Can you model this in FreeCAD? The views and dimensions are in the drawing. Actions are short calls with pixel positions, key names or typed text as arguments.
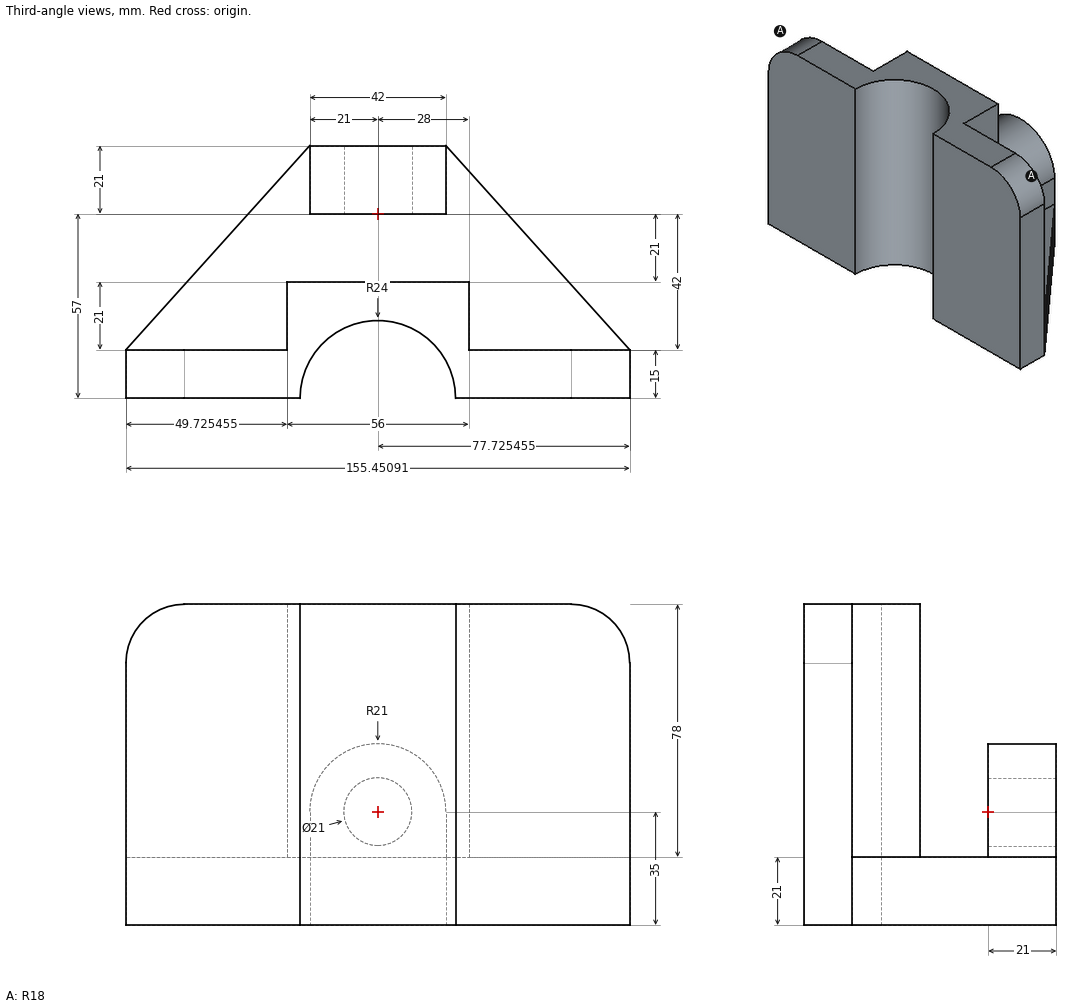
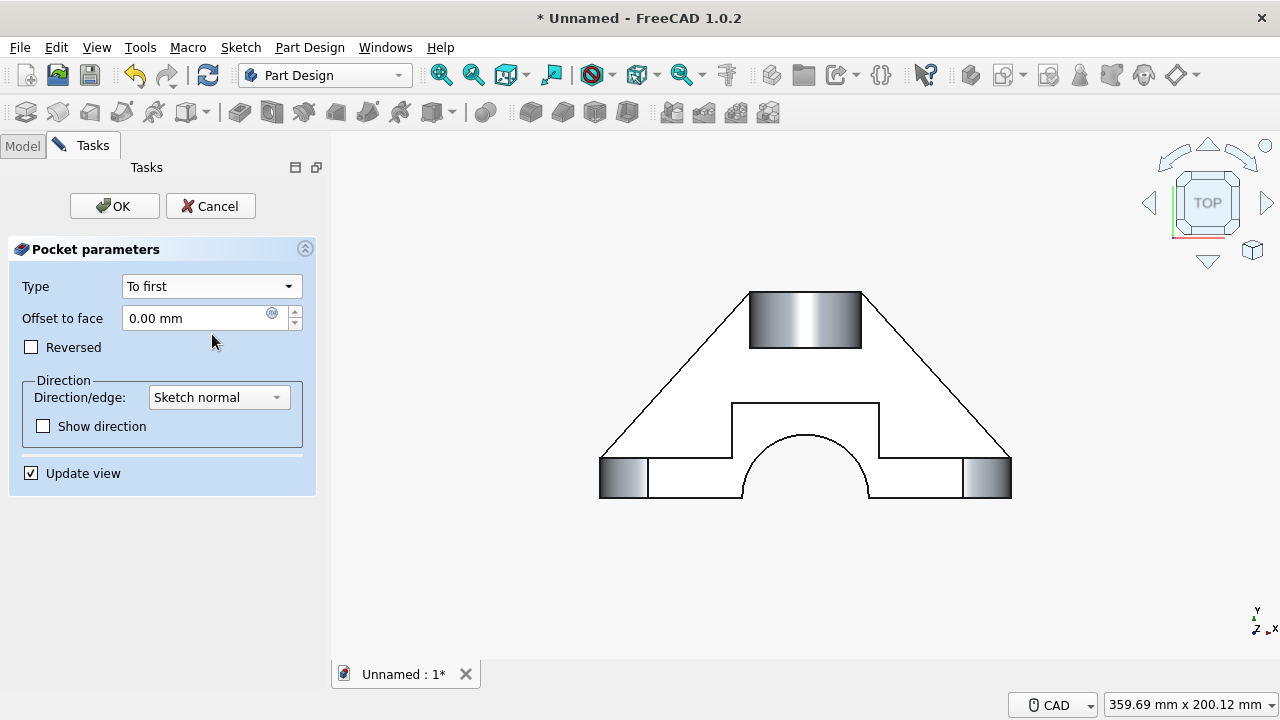
click(115, 206)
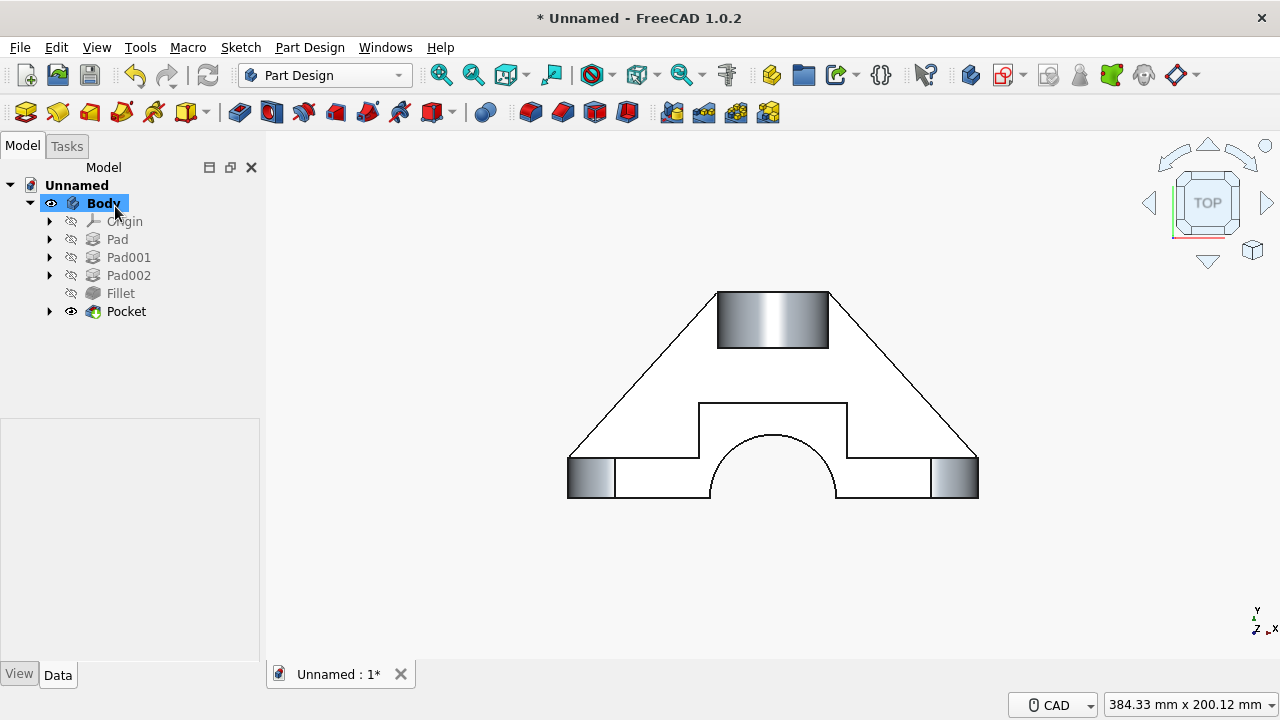
key(0)